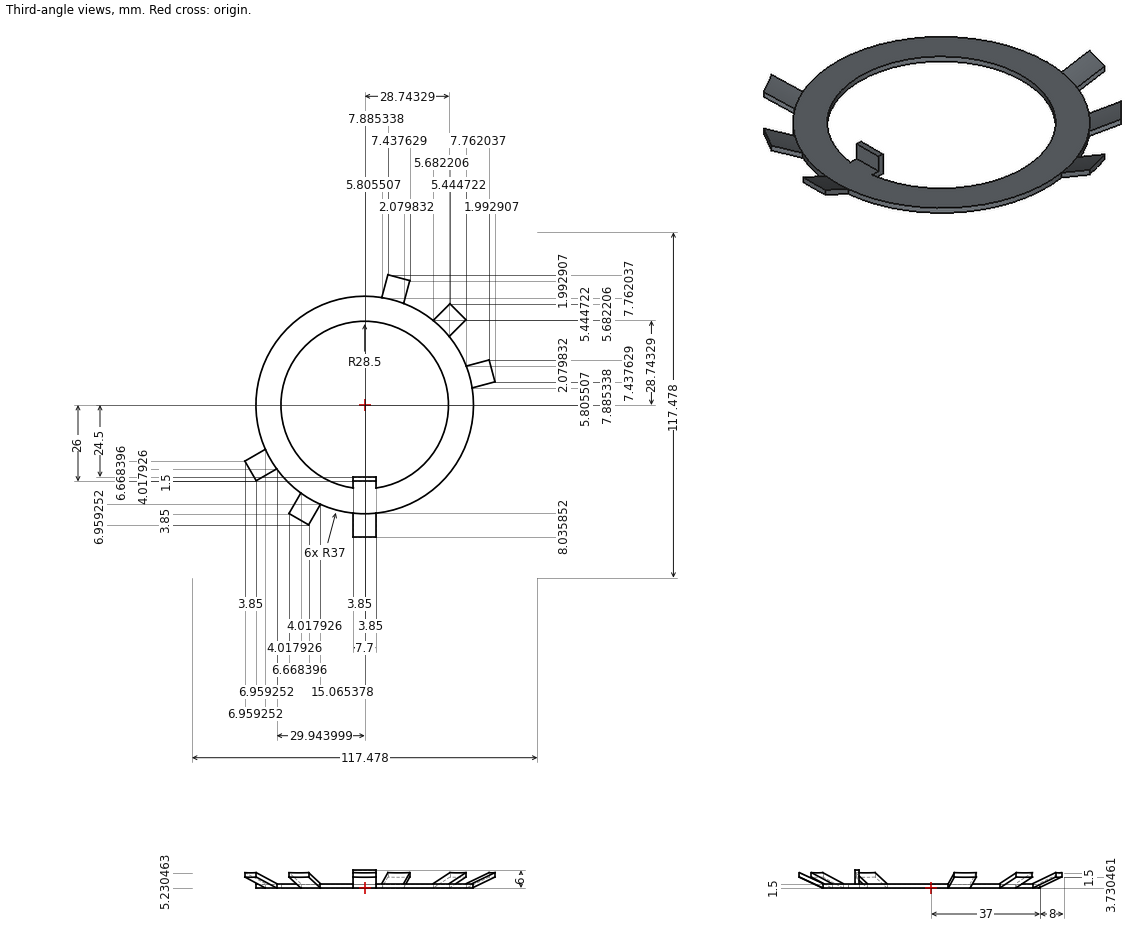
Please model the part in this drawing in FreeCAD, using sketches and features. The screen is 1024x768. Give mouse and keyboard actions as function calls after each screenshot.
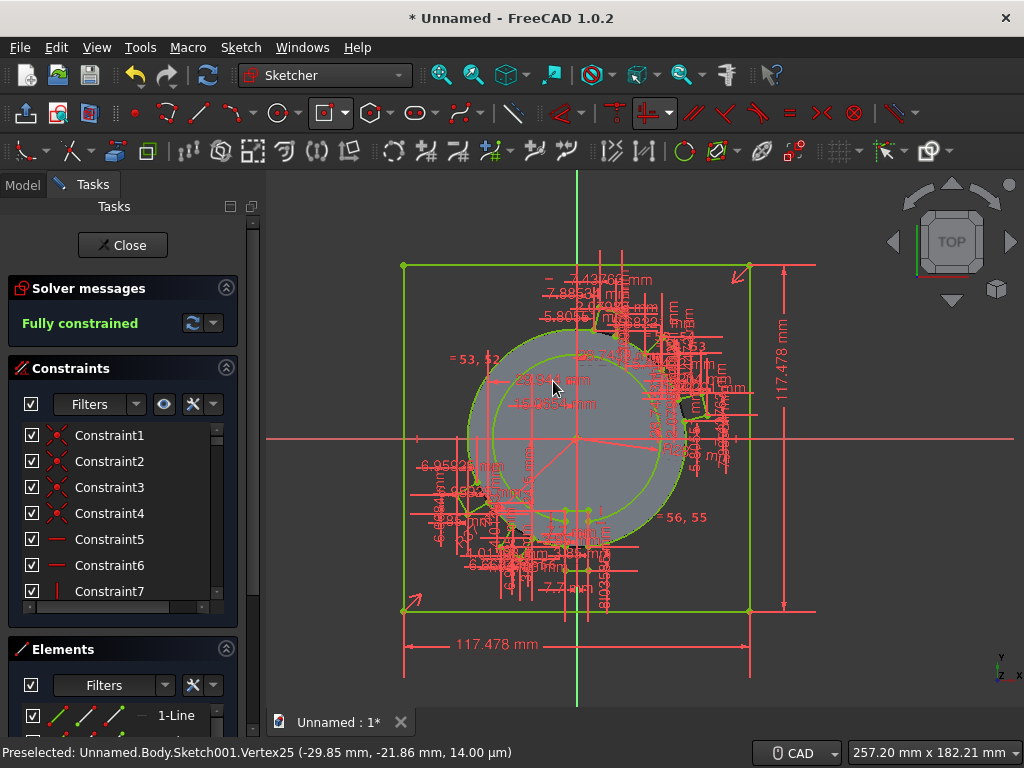
click(123, 245)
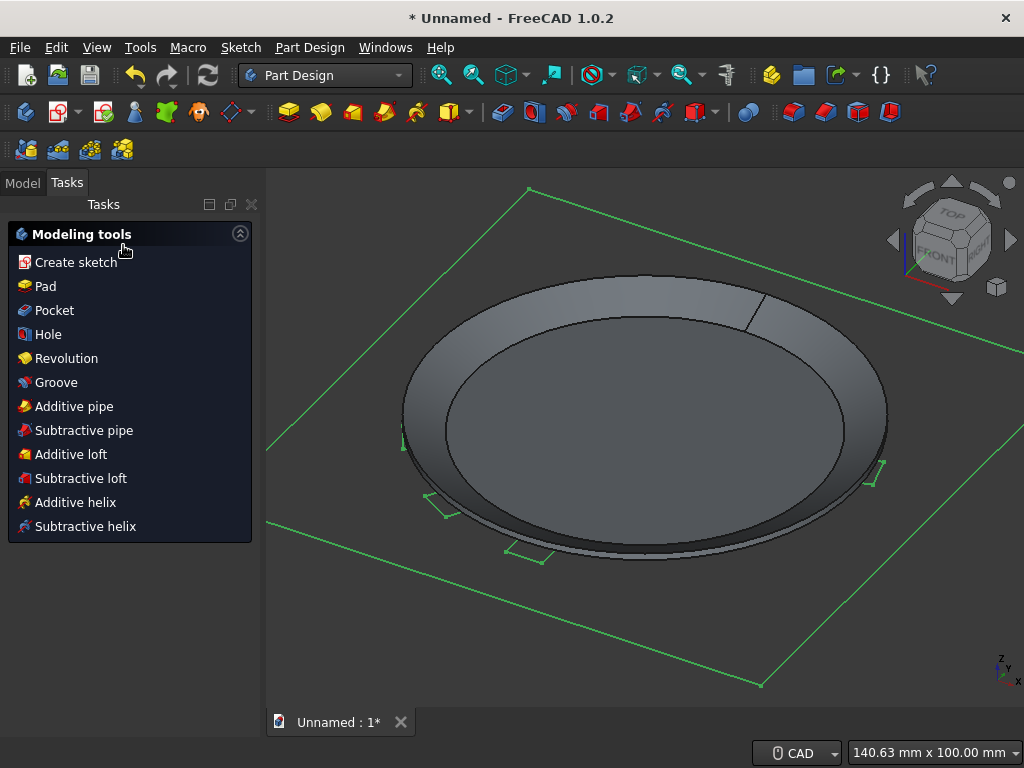
click(504, 112)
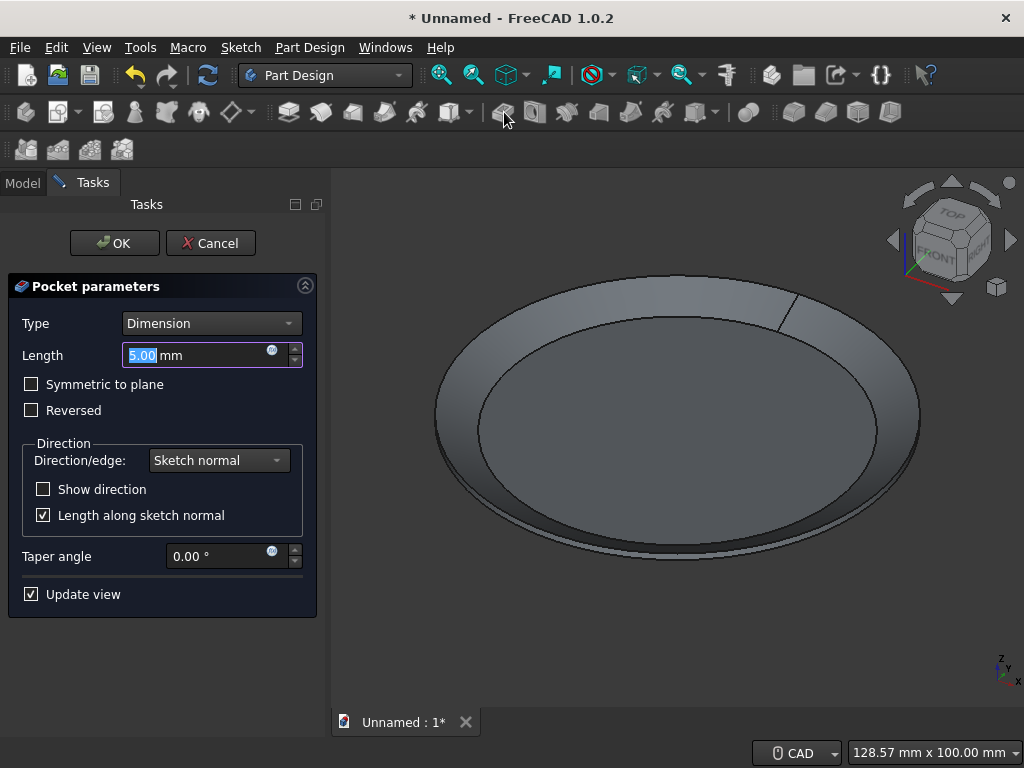
text(5.230463)
key(Tab)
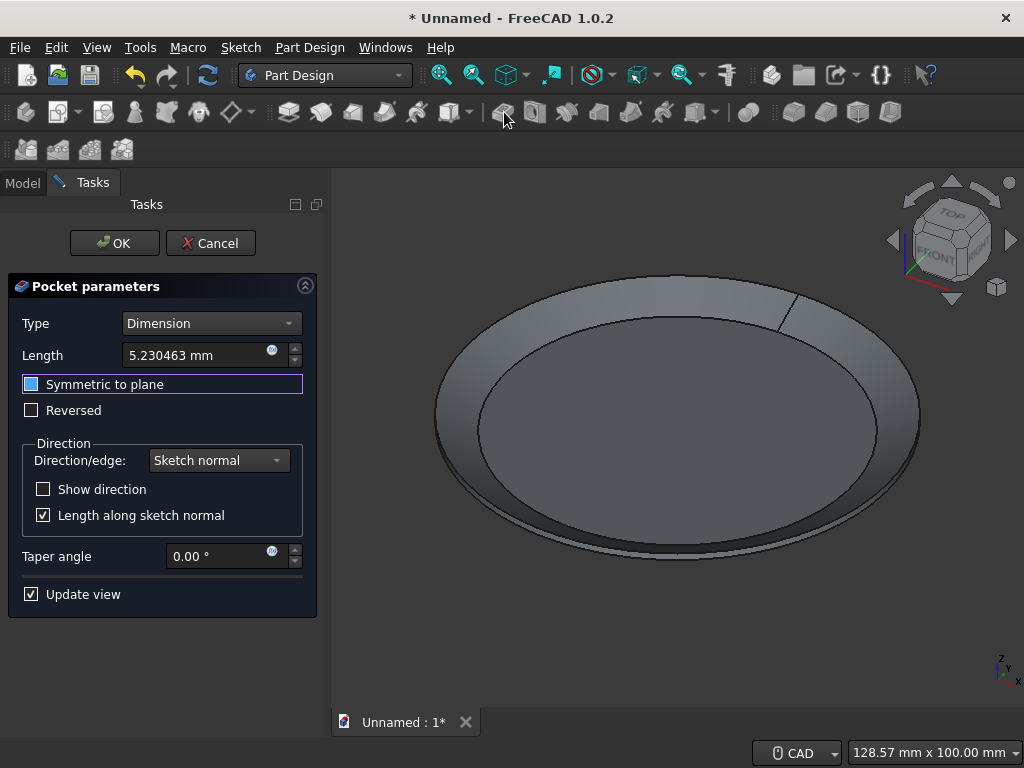
click(30, 410)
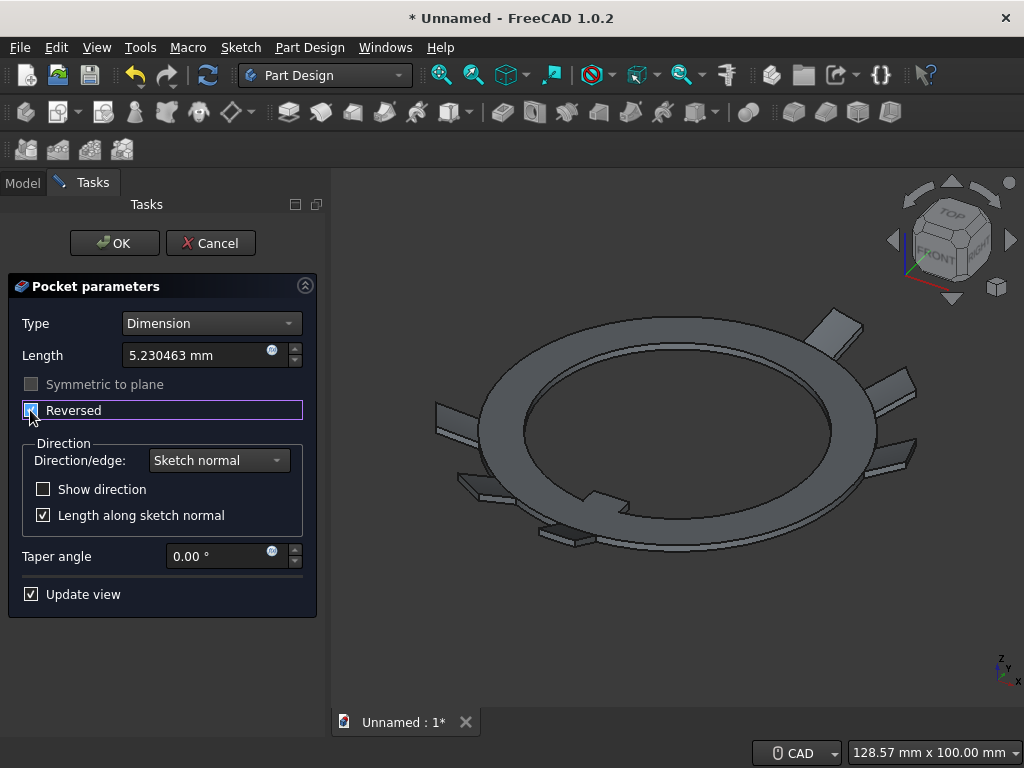
click(115, 243)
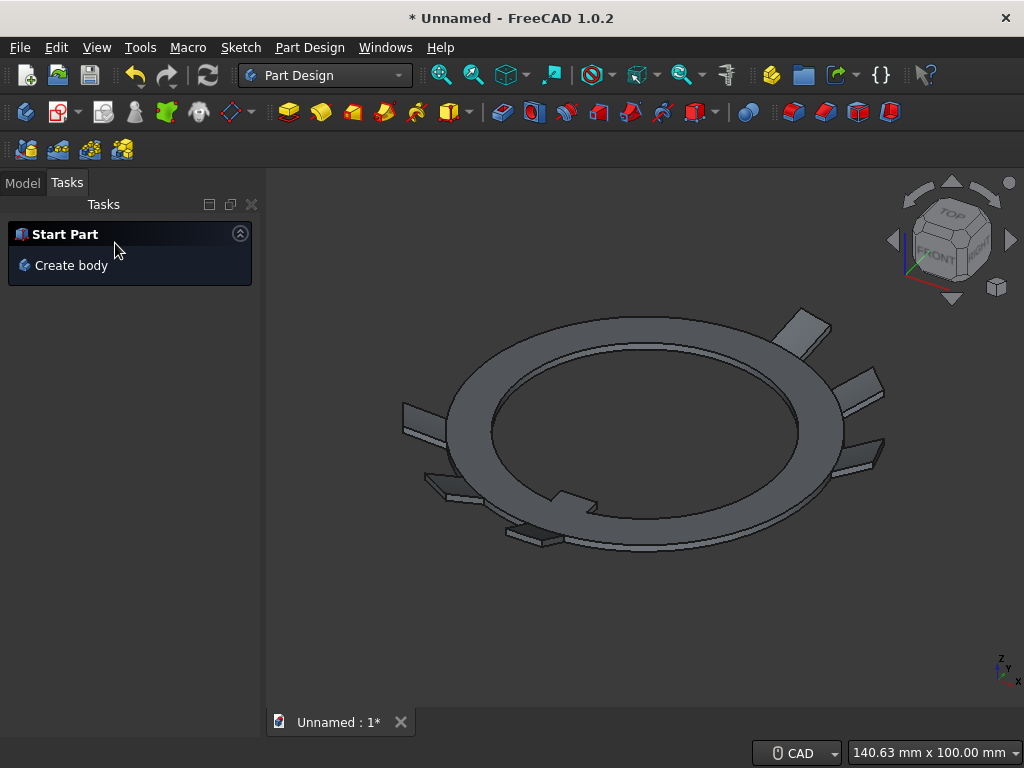
click(58, 112)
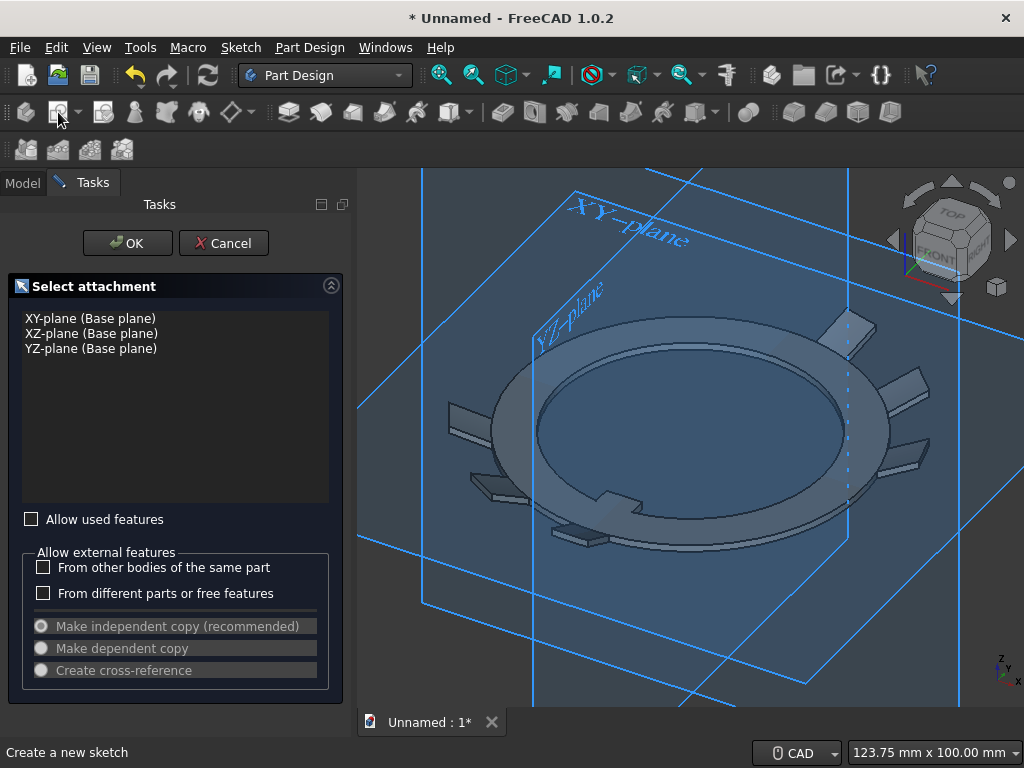
click(82, 318)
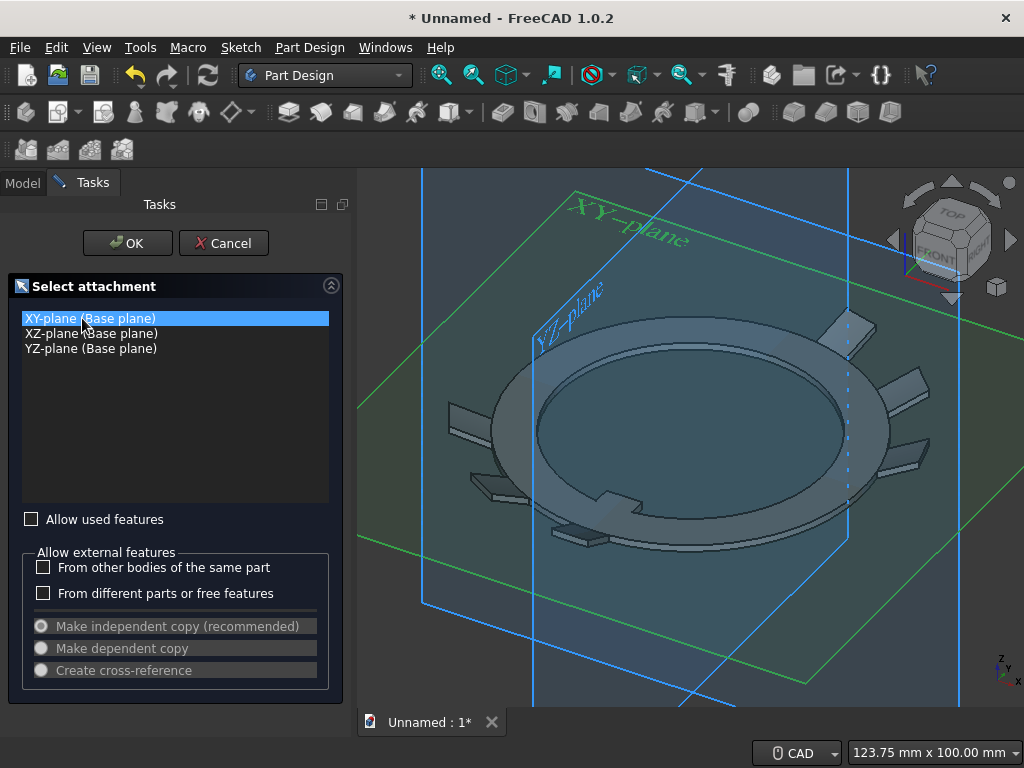
click(128, 243)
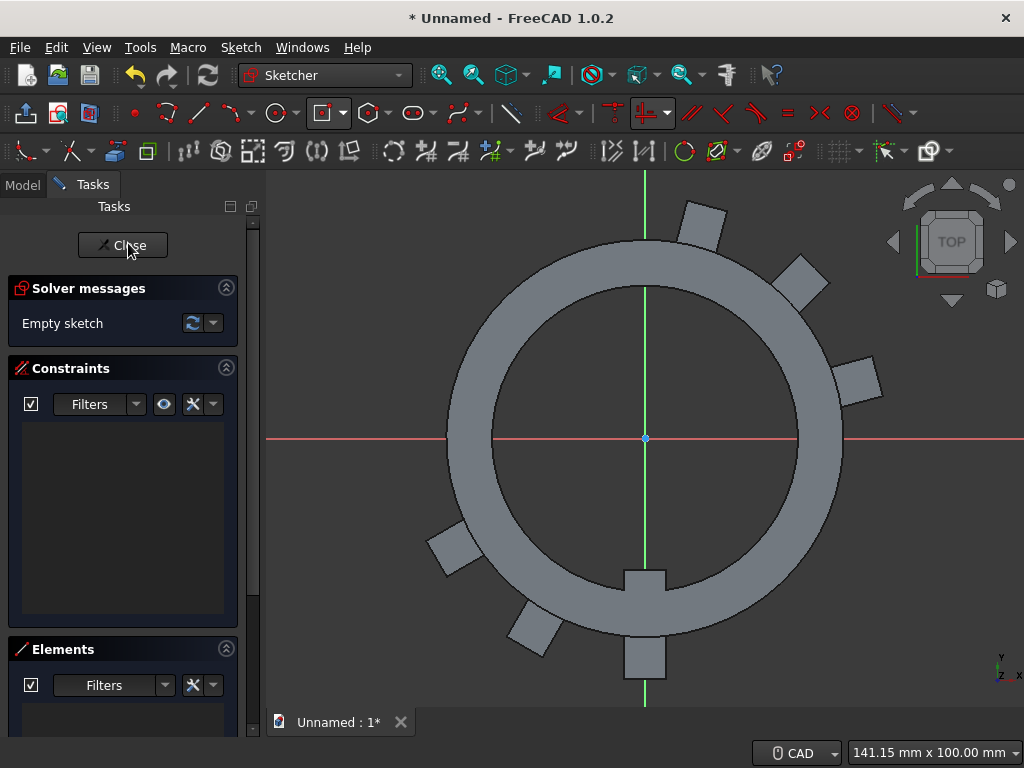
click(90, 114)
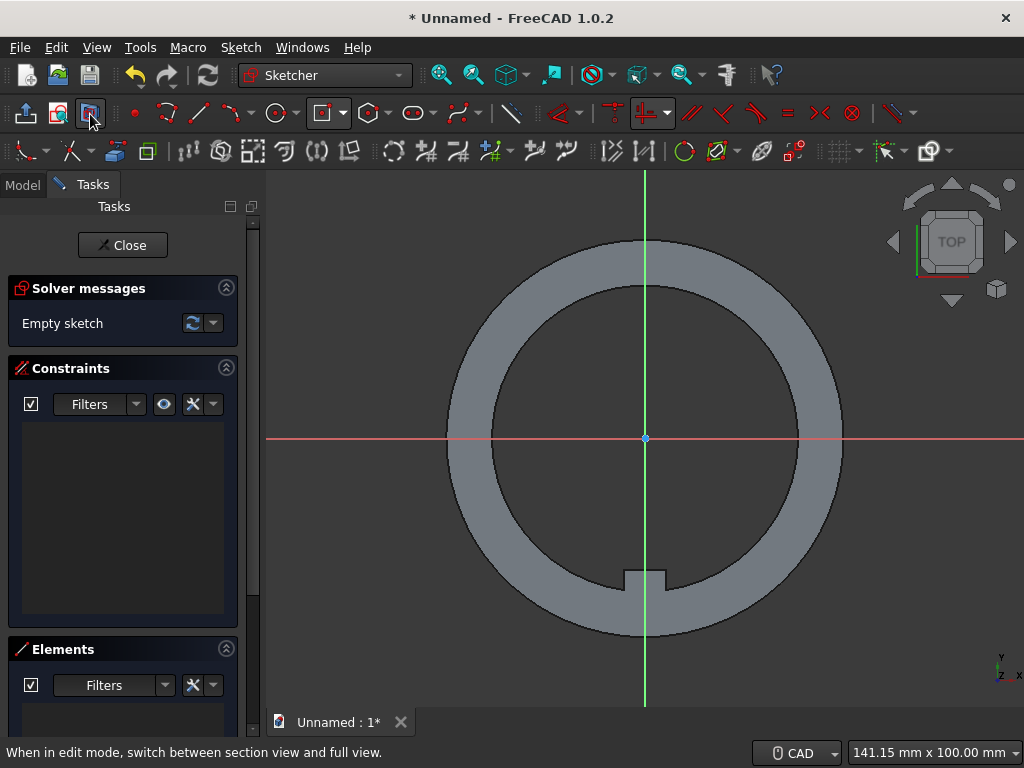
scroll(654, 591, up, 11)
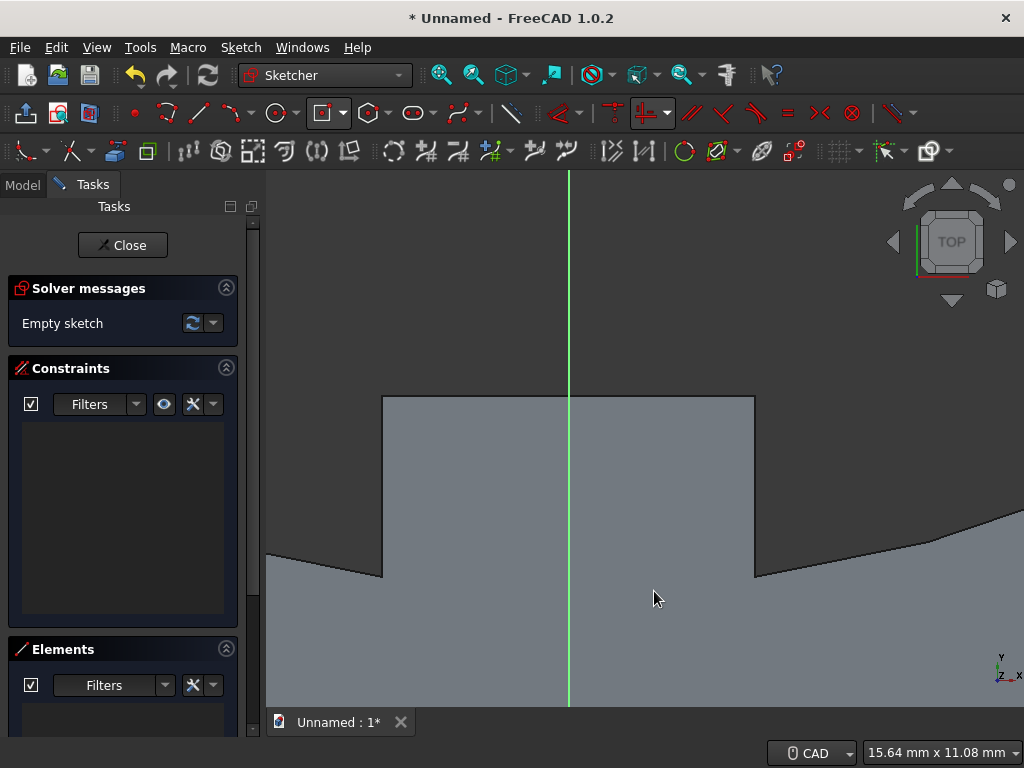
key(g)
key(r)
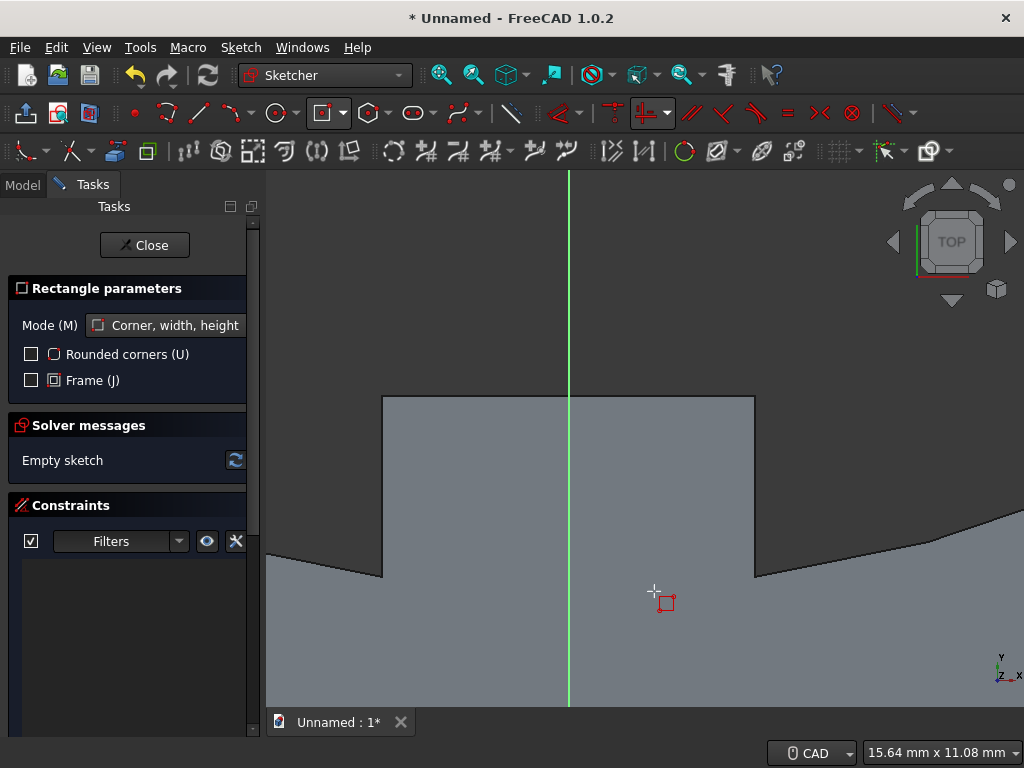
click(382, 396)
click(755, 468)
key(Escape)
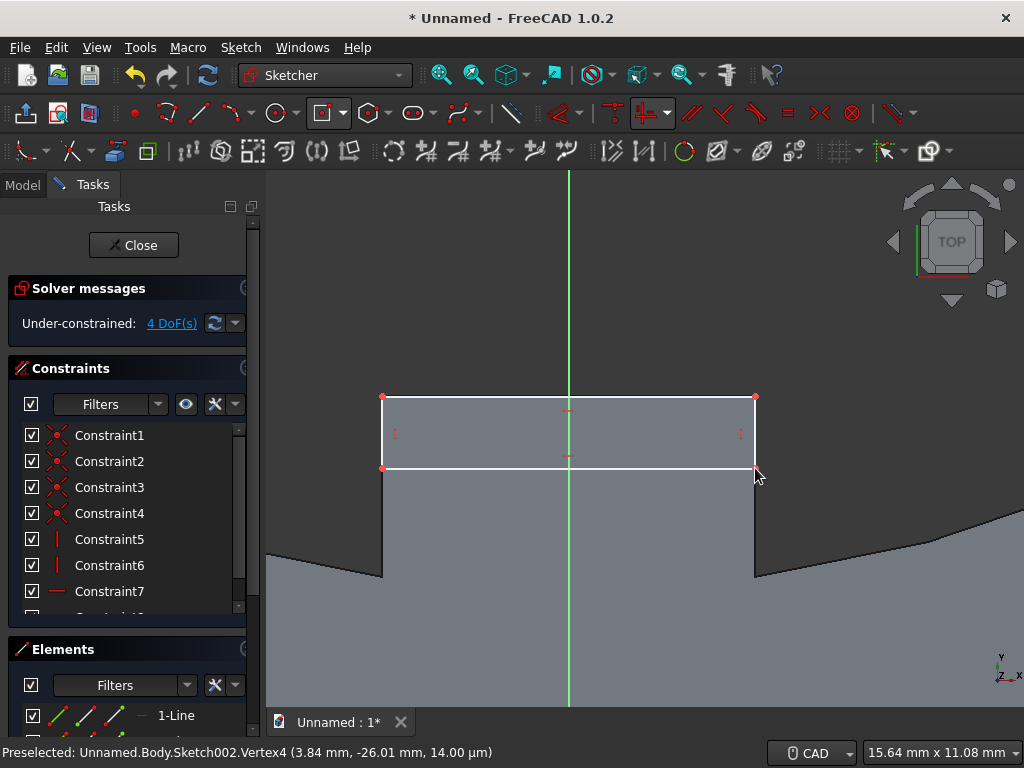
click(558, 114)